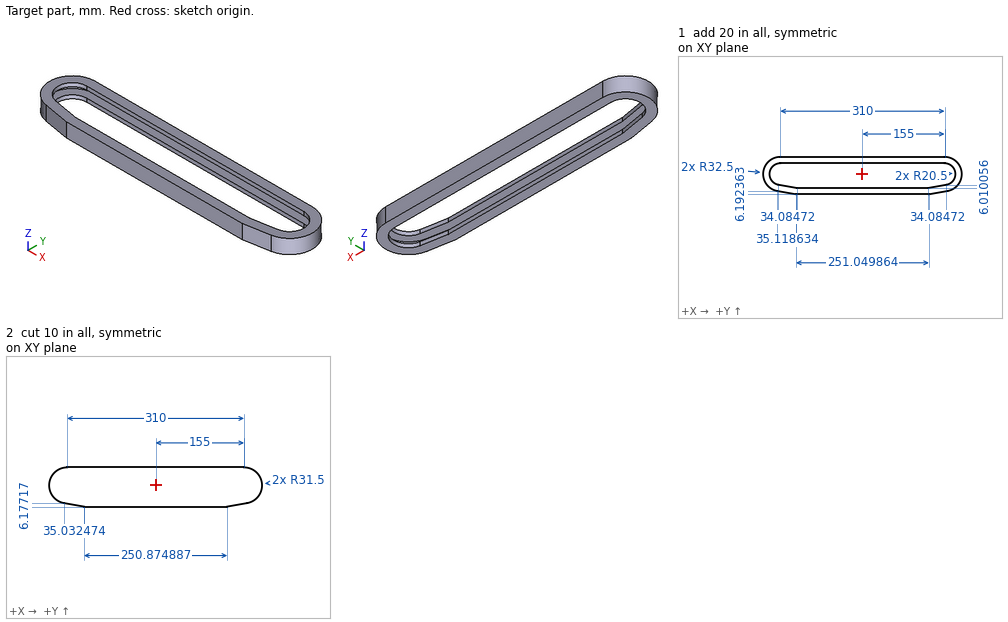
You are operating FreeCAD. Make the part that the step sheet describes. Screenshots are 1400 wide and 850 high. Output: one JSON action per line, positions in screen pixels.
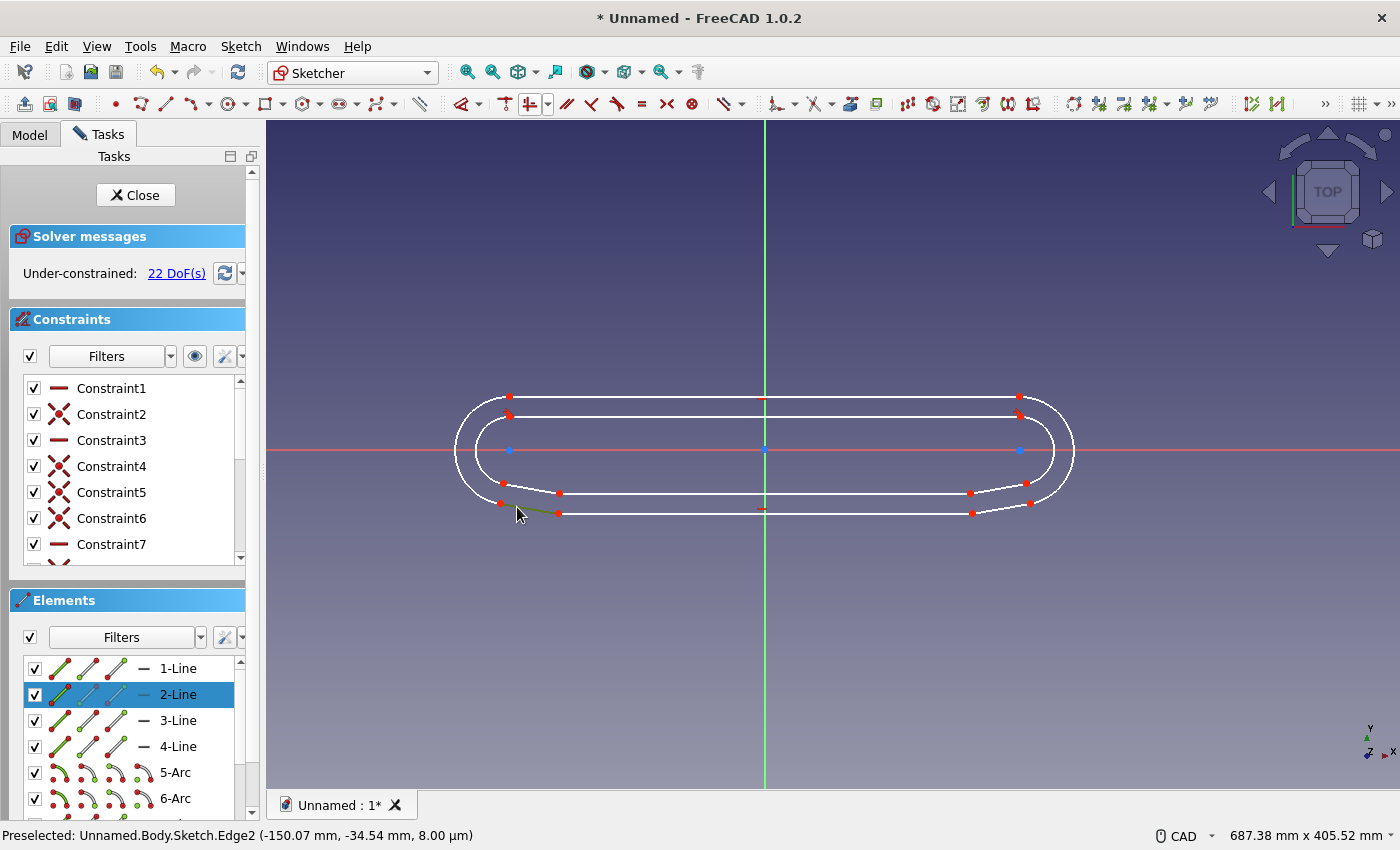
{"action": "left_click", "coordinate": [467, 417]}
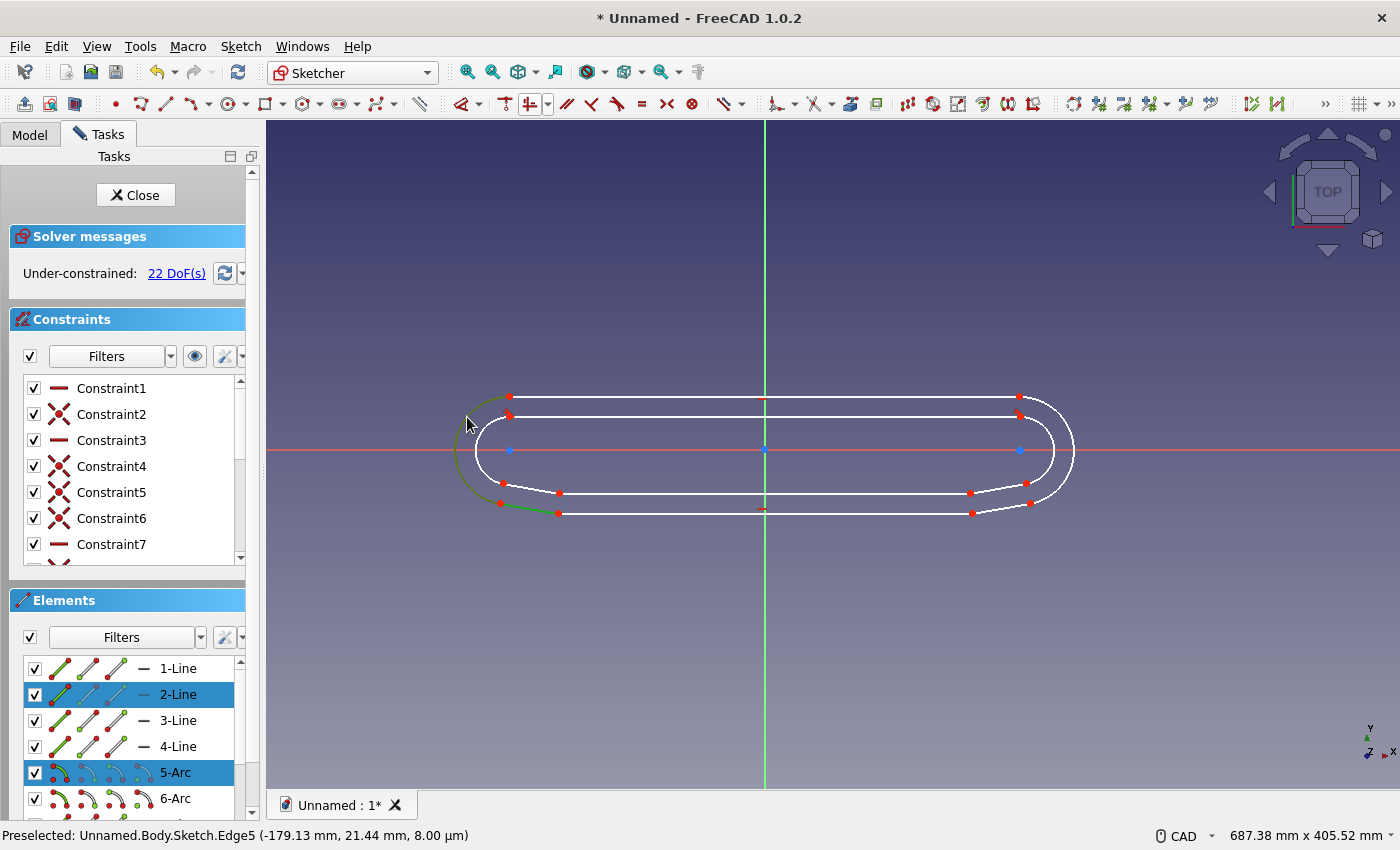
{"action": "left_click", "coordinate": [617, 104]}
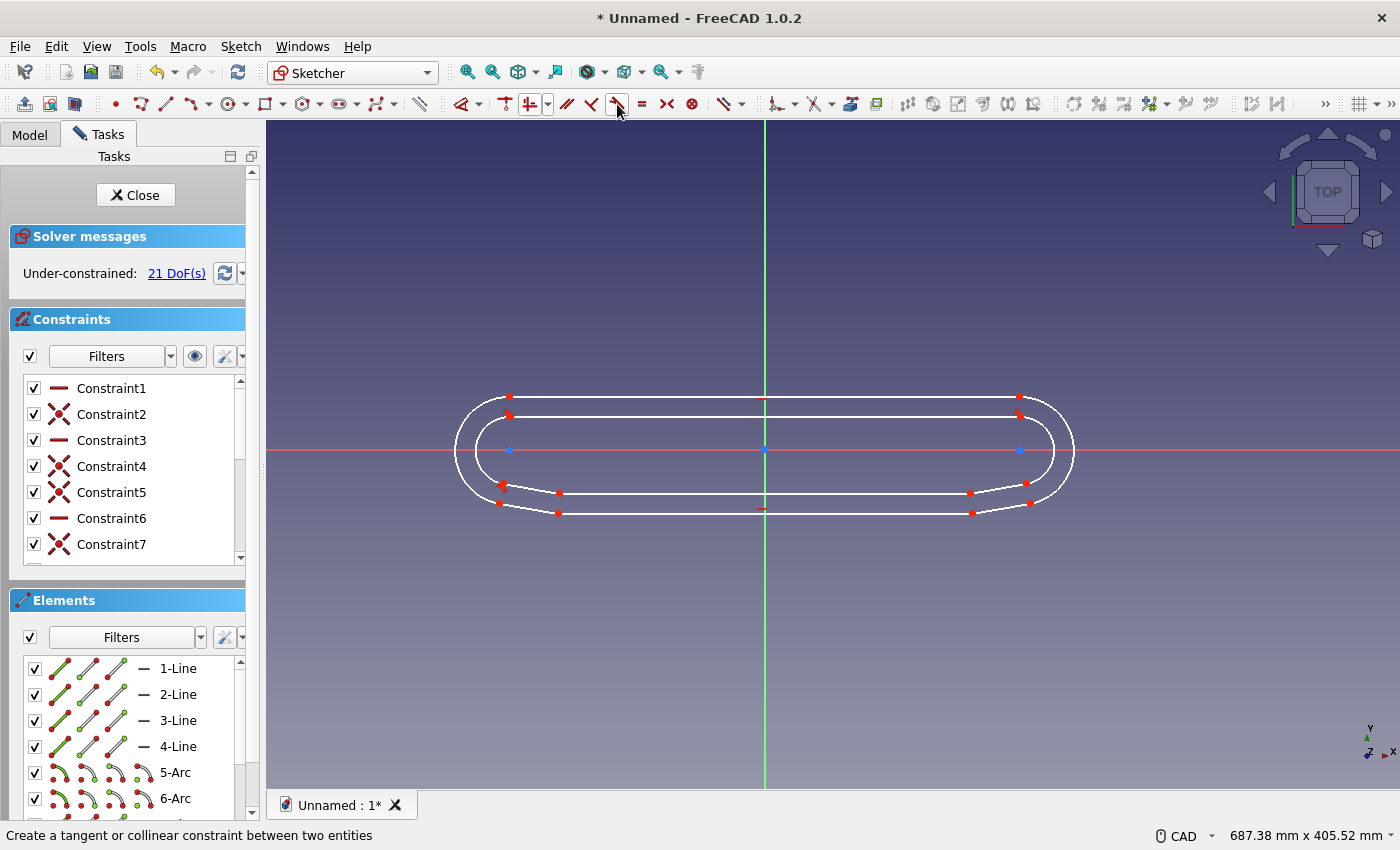
{"action": "left_click", "coordinate": [989, 511]}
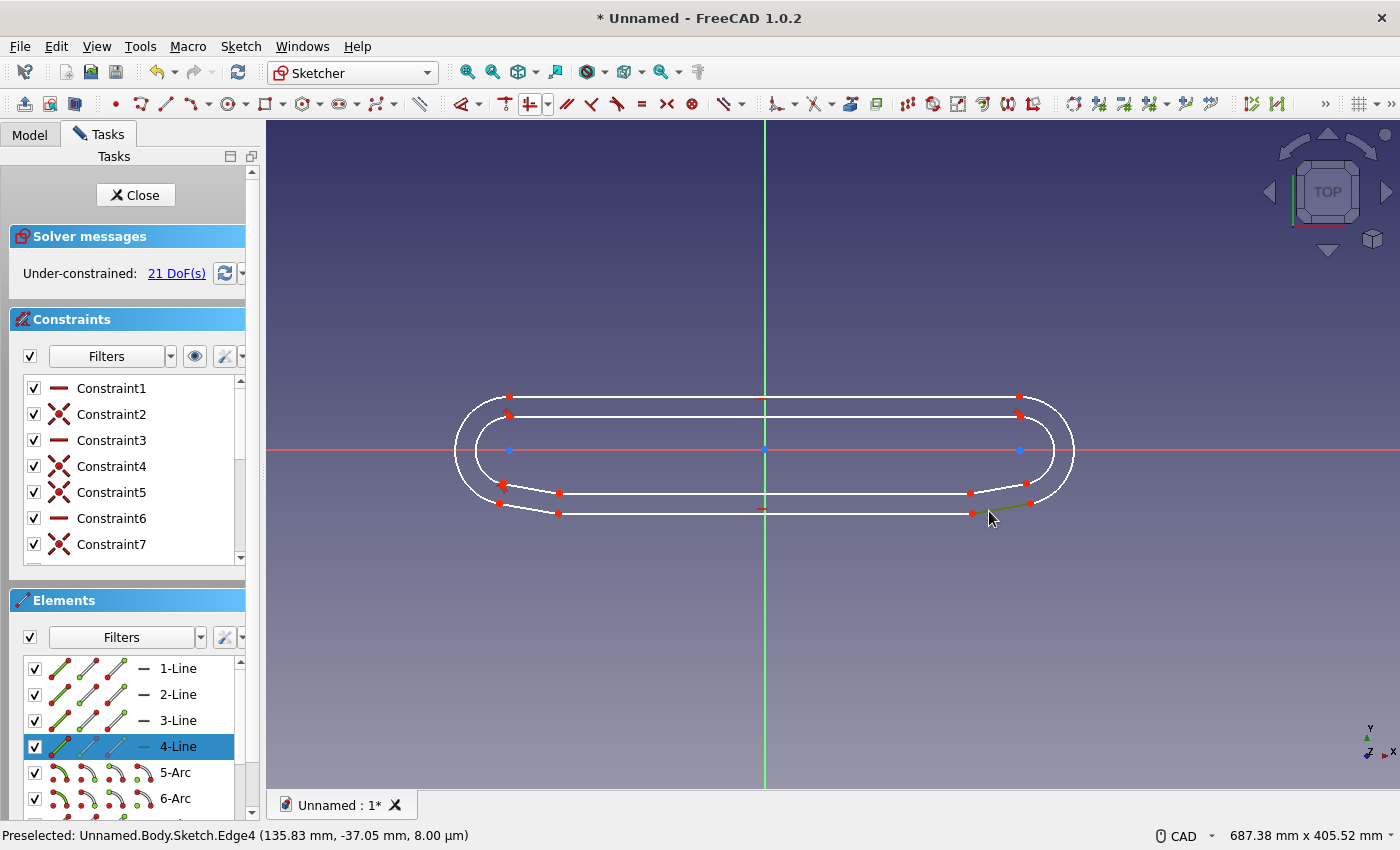
{"action": "left_click", "coordinate": [1067, 477]}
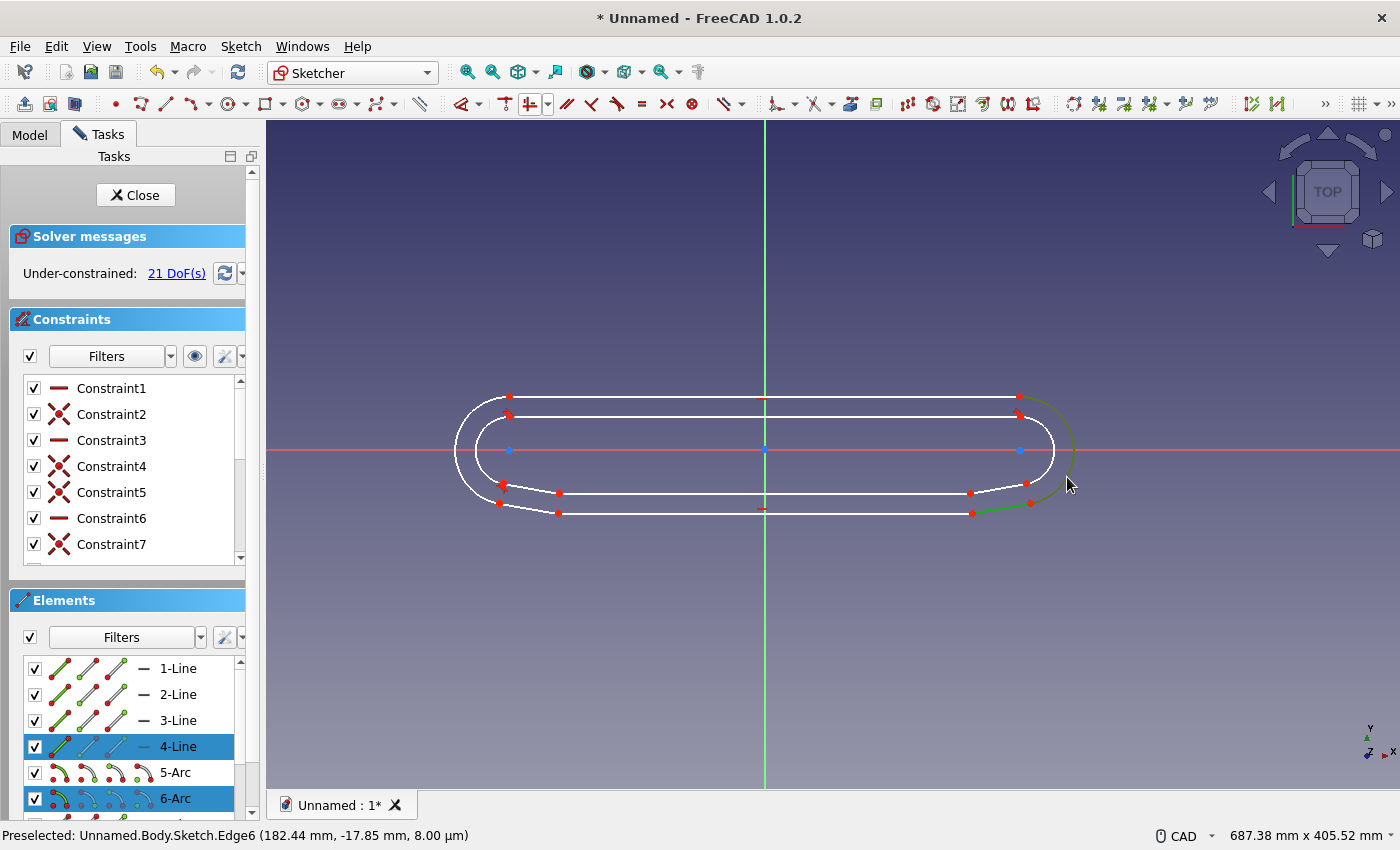
{"action": "left_click", "coordinate": [617, 104]}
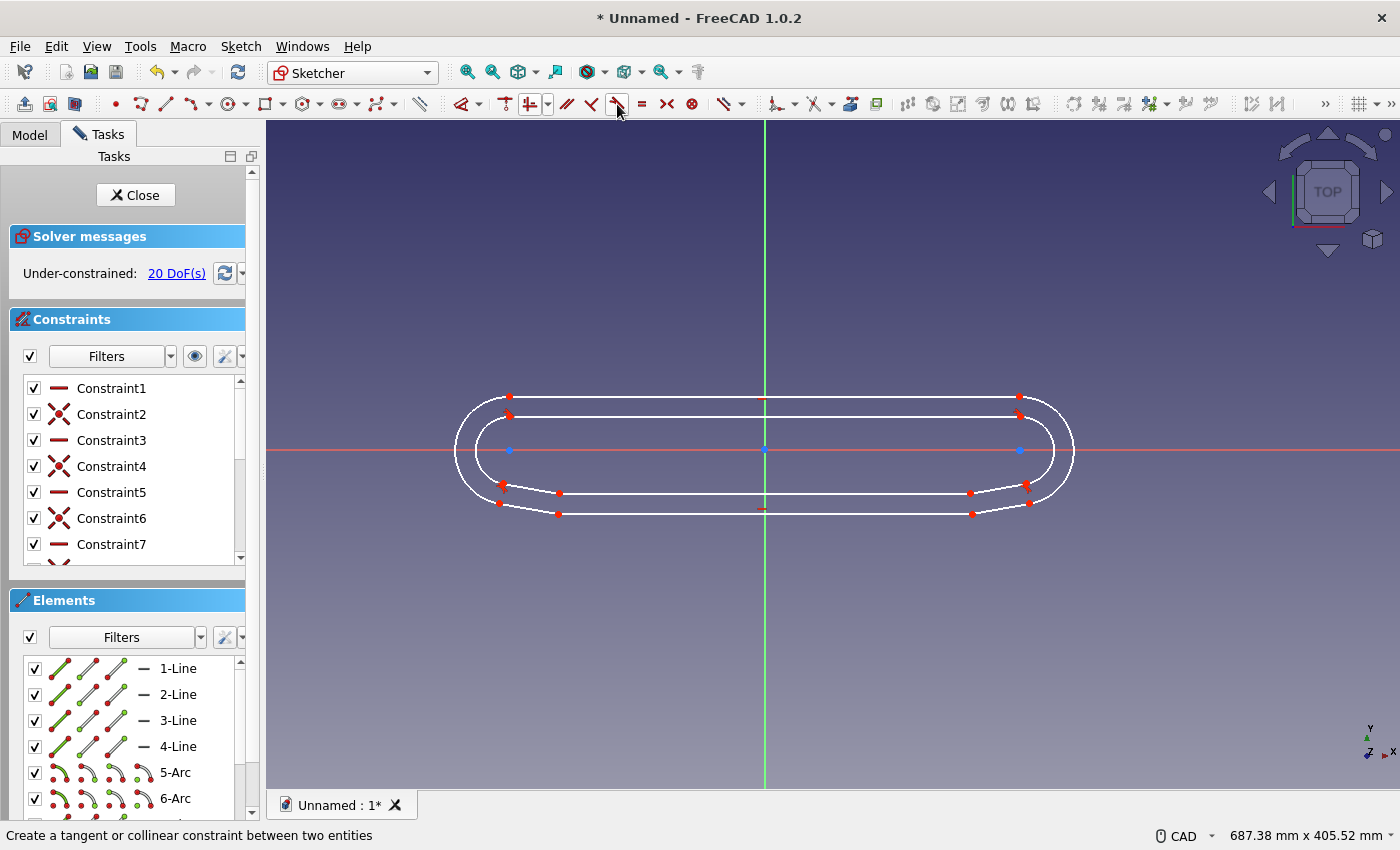
{"action": "left_click", "coordinate": [662, 417]}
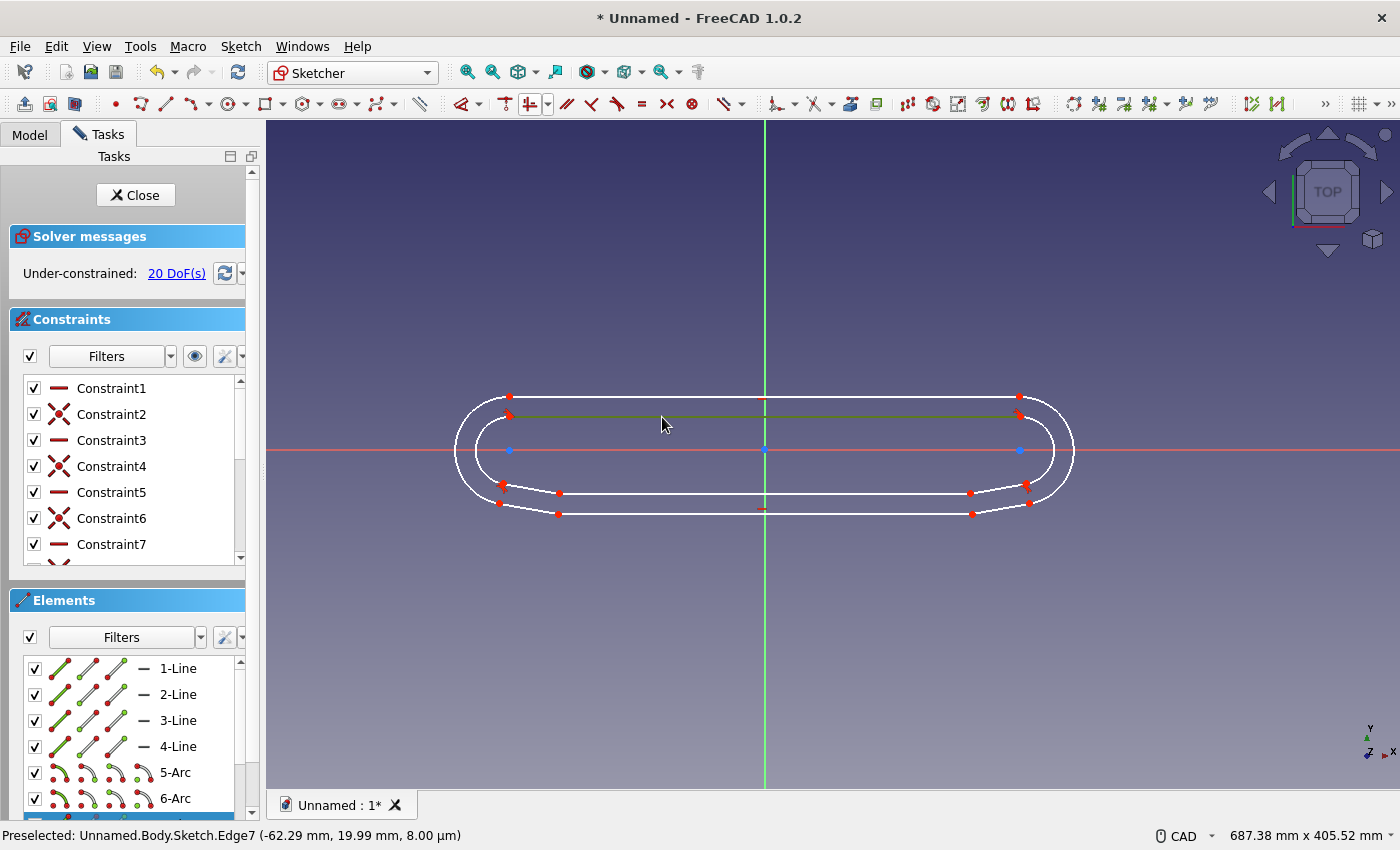
{"action": "left_click", "coordinate": [1050, 467]}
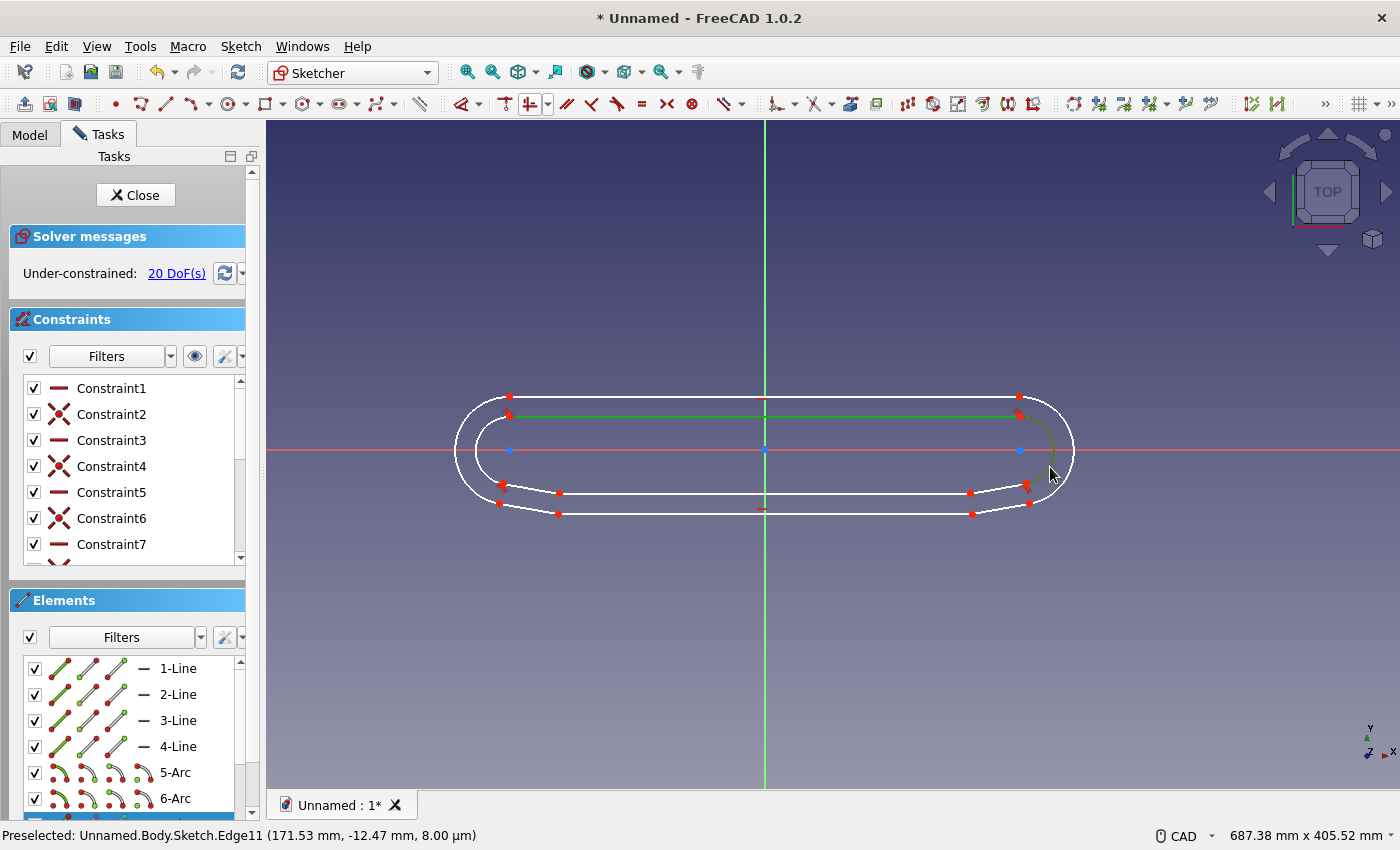
{"action": "key", "text": "t"}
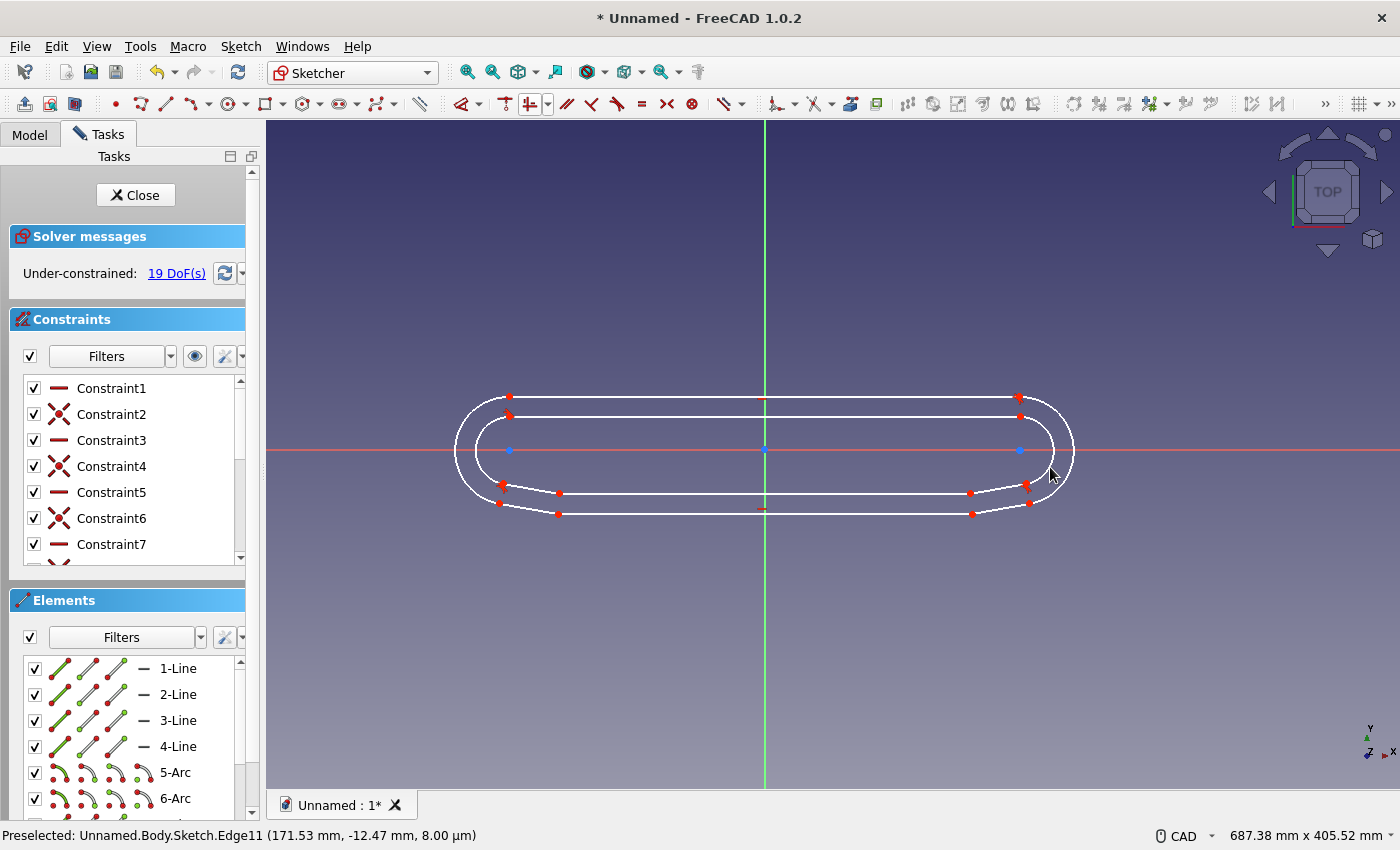
{"action": "left_click", "coordinate": [662, 417]}